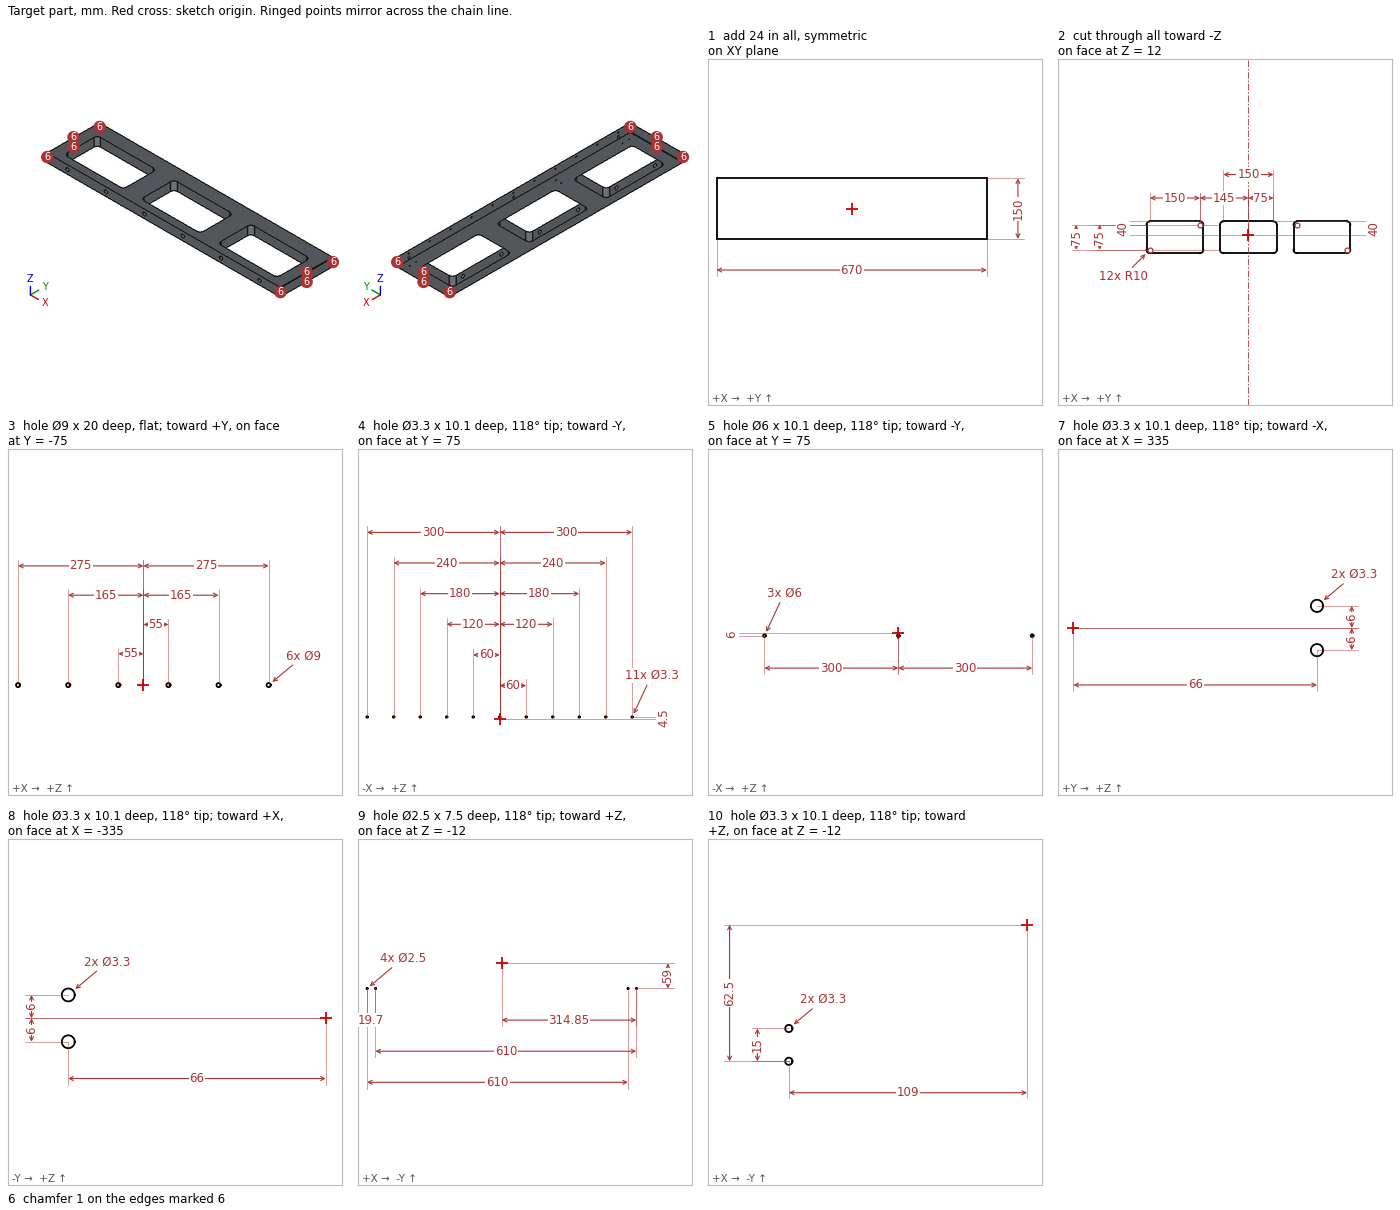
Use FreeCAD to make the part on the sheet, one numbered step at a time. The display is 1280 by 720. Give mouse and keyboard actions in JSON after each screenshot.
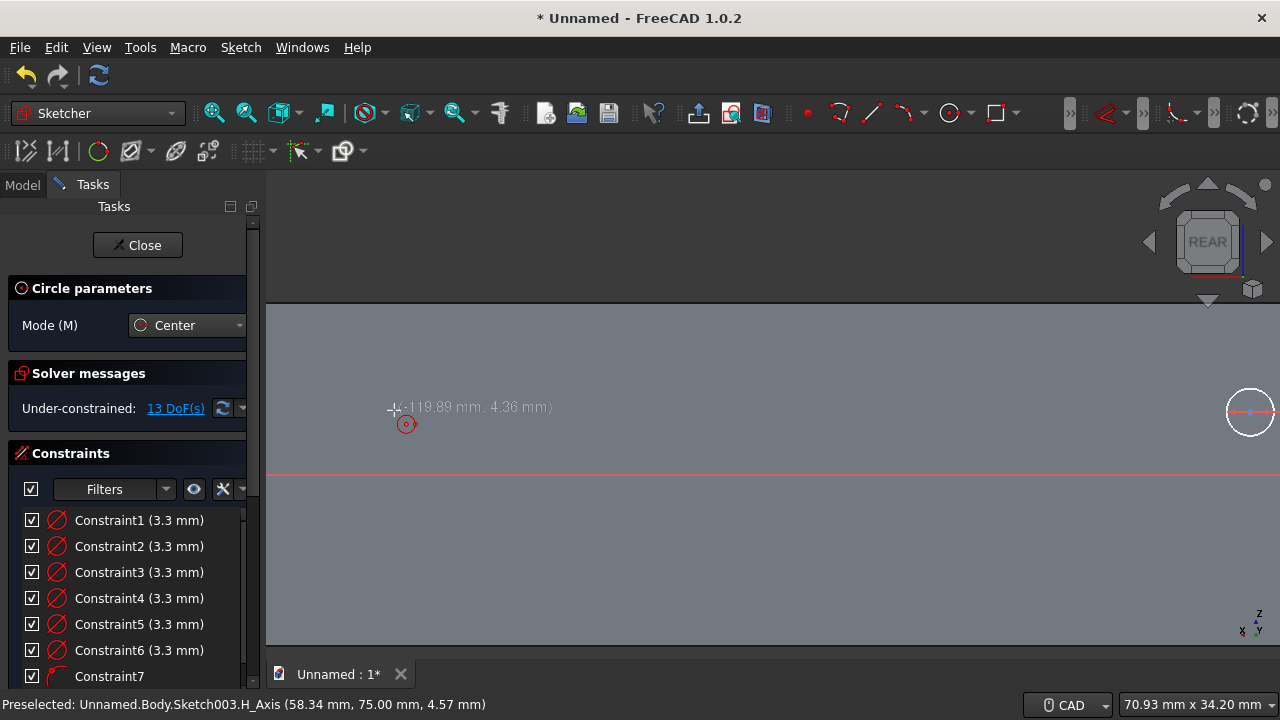
{"action": "scroll", "coordinate": [614, 413], "scroll_direction": "down", "scroll_amount": 14}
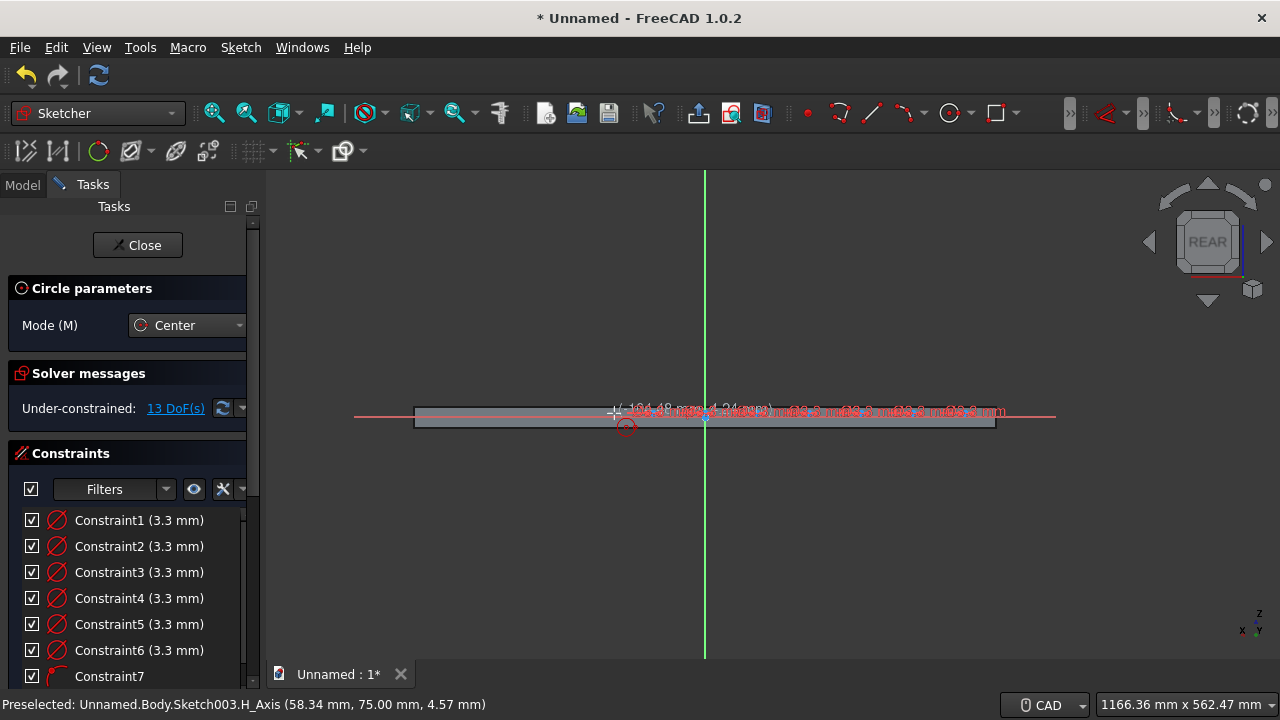
{"action": "scroll", "coordinate": [601, 413], "scroll_direction": "up", "scroll_amount": 8}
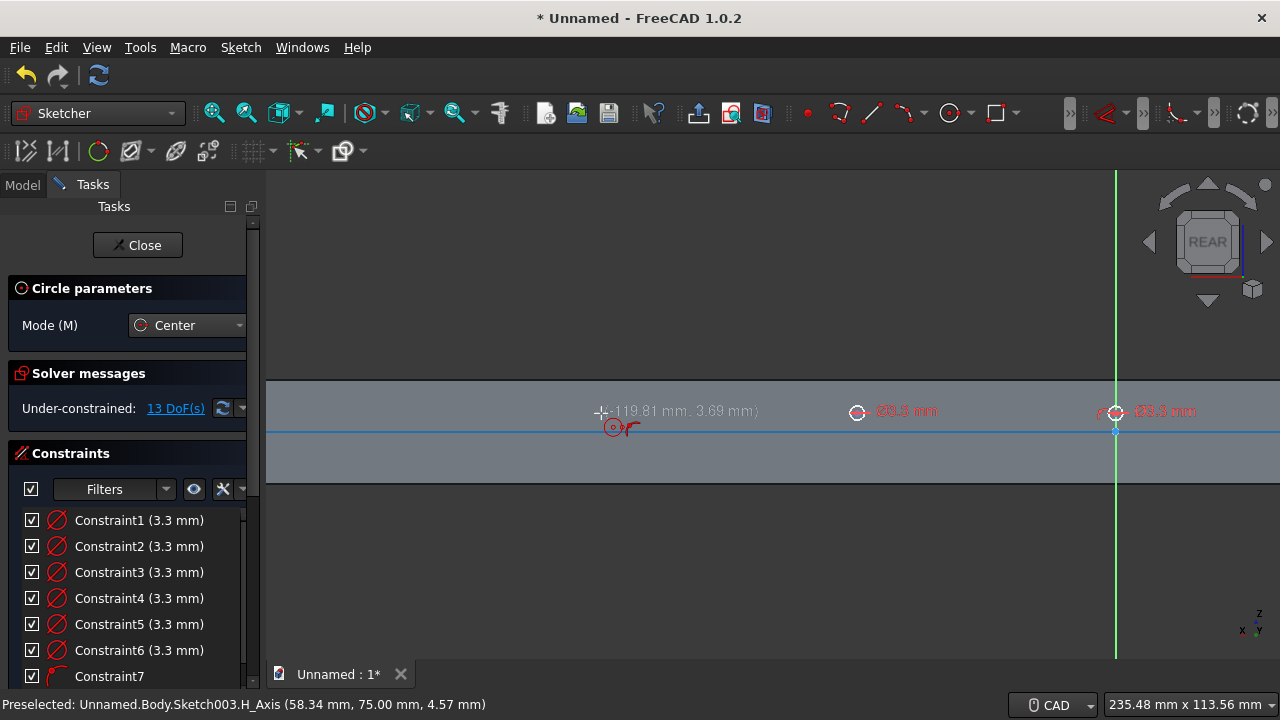
{"action": "left_click", "coordinate": [599, 413]}
{"action": "mouse_move", "coordinate": [604, 407]}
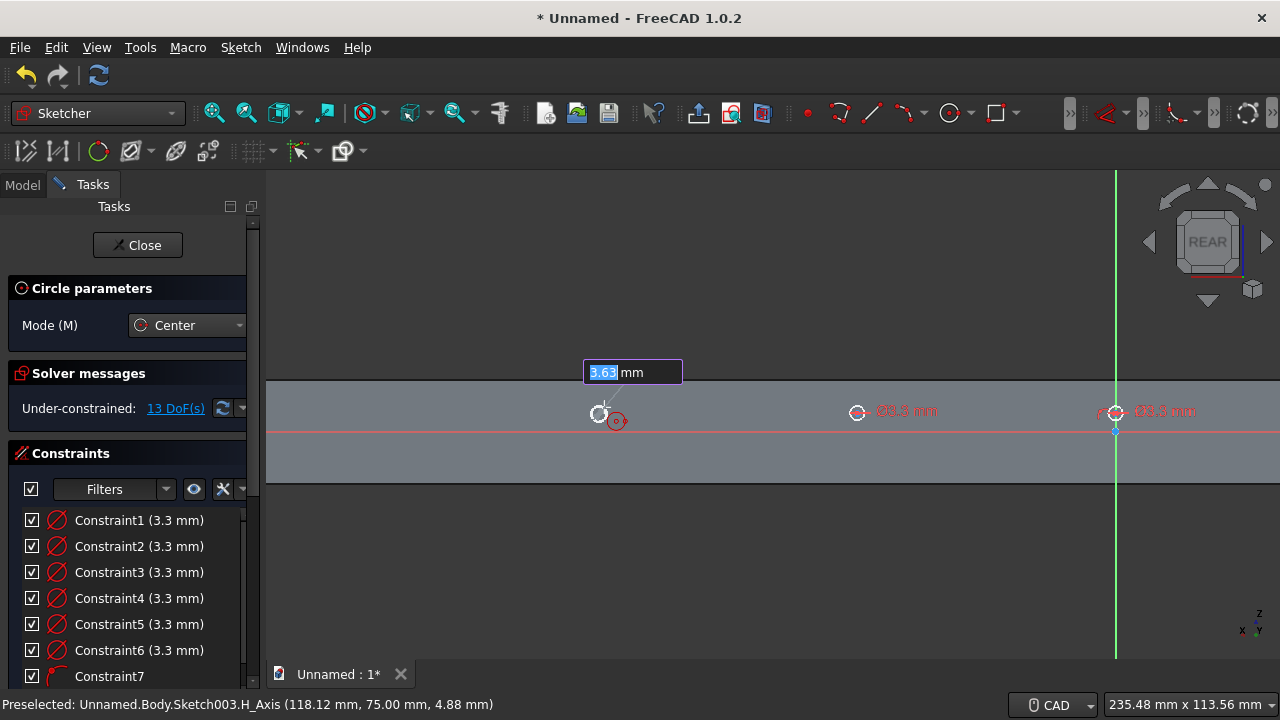
{"action": "type", "text": "3.3"}
{"action": "key", "text": "Return"}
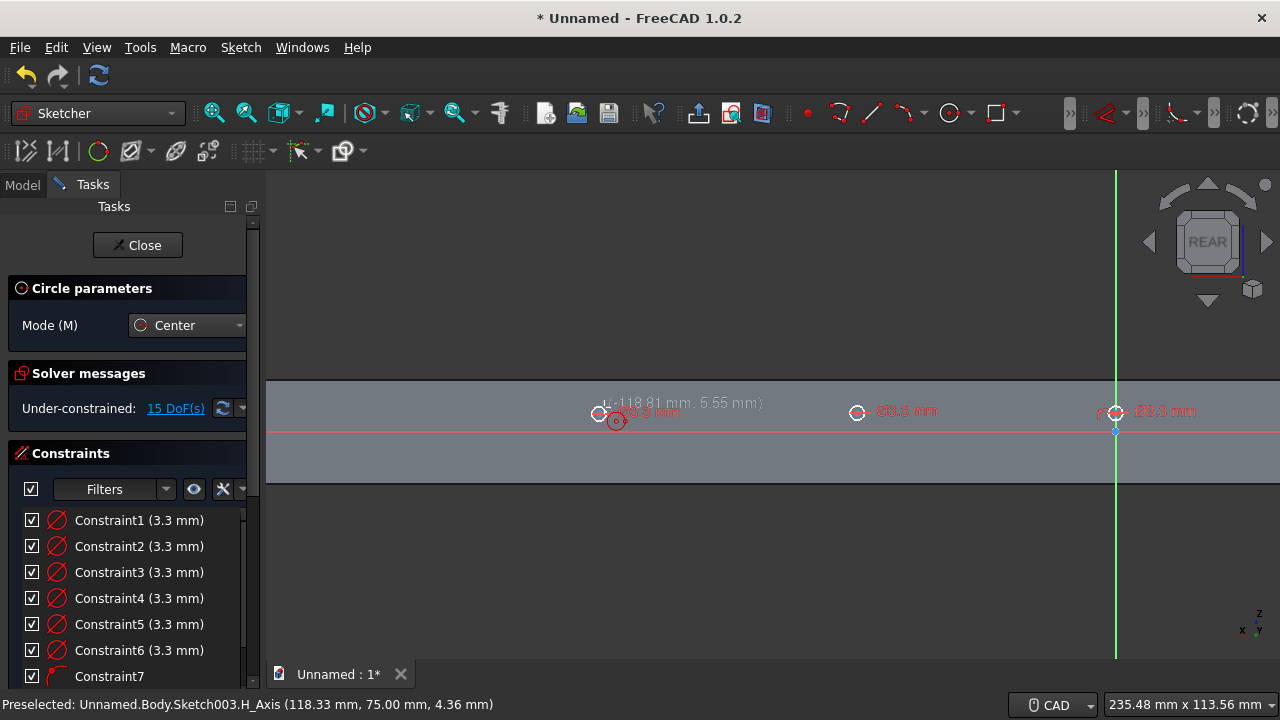
{"action": "scroll", "coordinate": [341, 413], "scroll_direction": "up", "scroll_amount": 6}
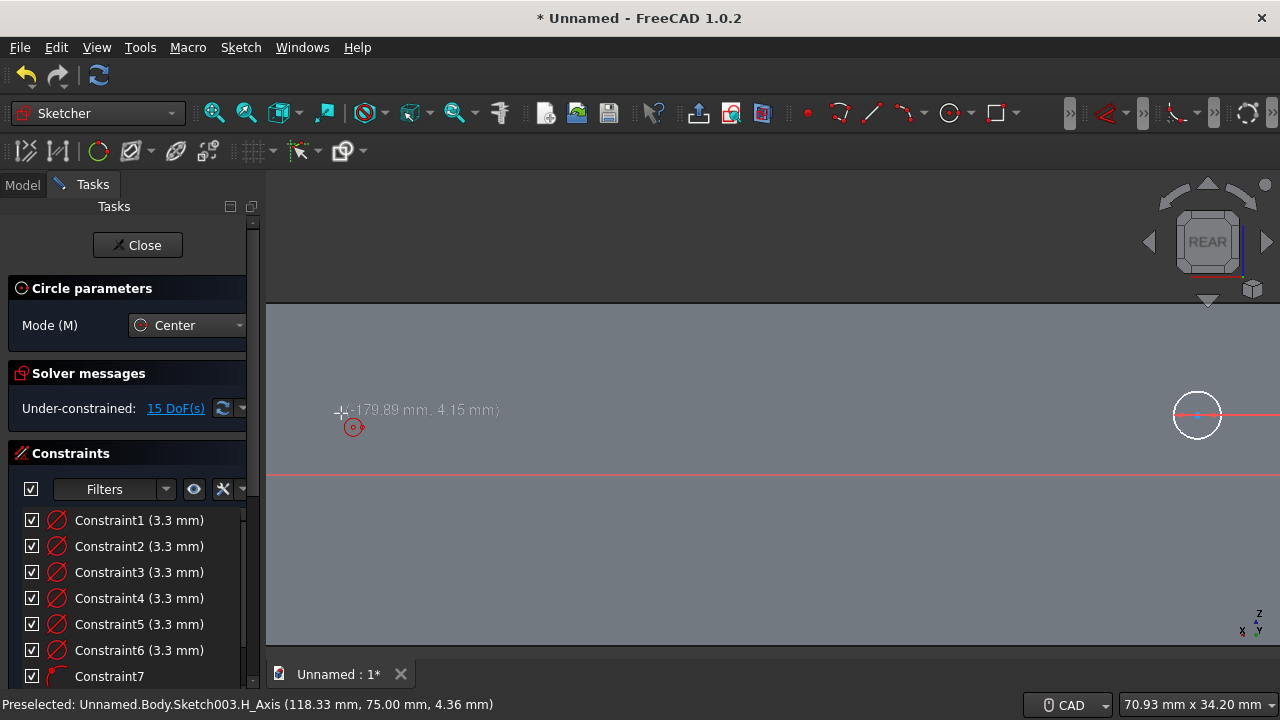
{"action": "scroll", "coordinate": [562, 413], "scroll_direction": "down", "scroll_amount": 14}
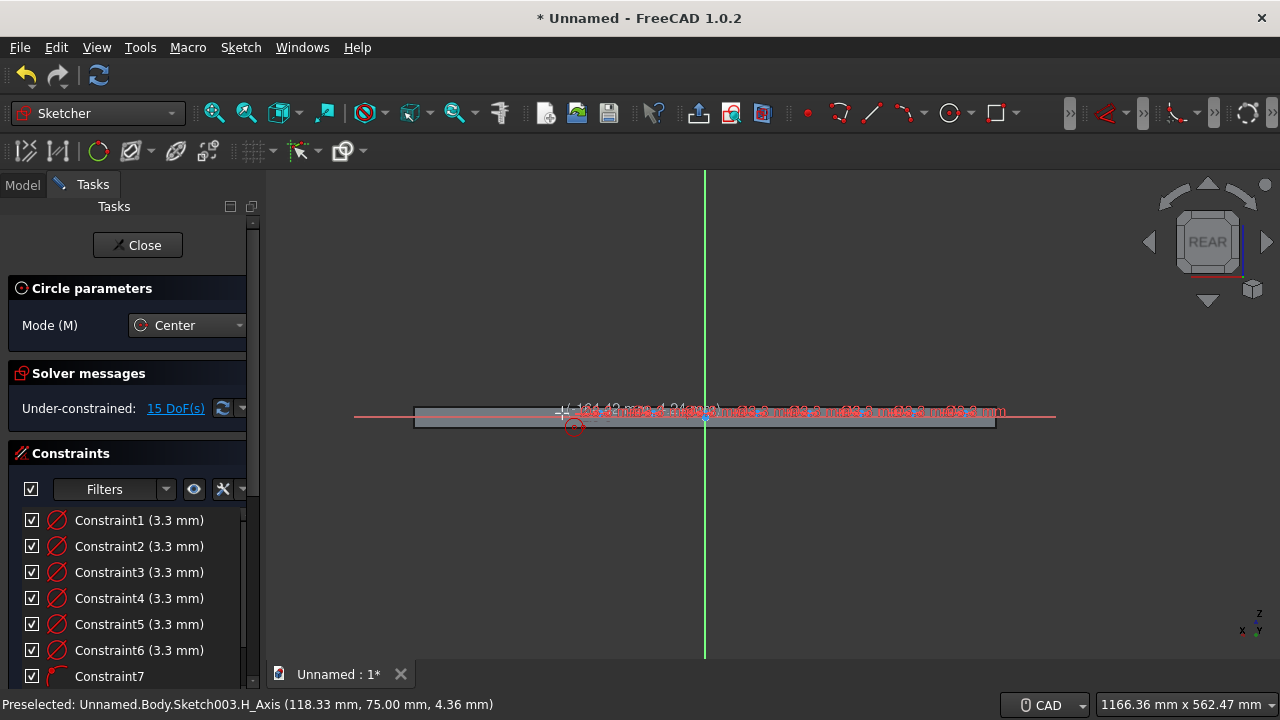
{"action": "scroll", "coordinate": [549, 413], "scroll_direction": "up", "scroll_amount": 8}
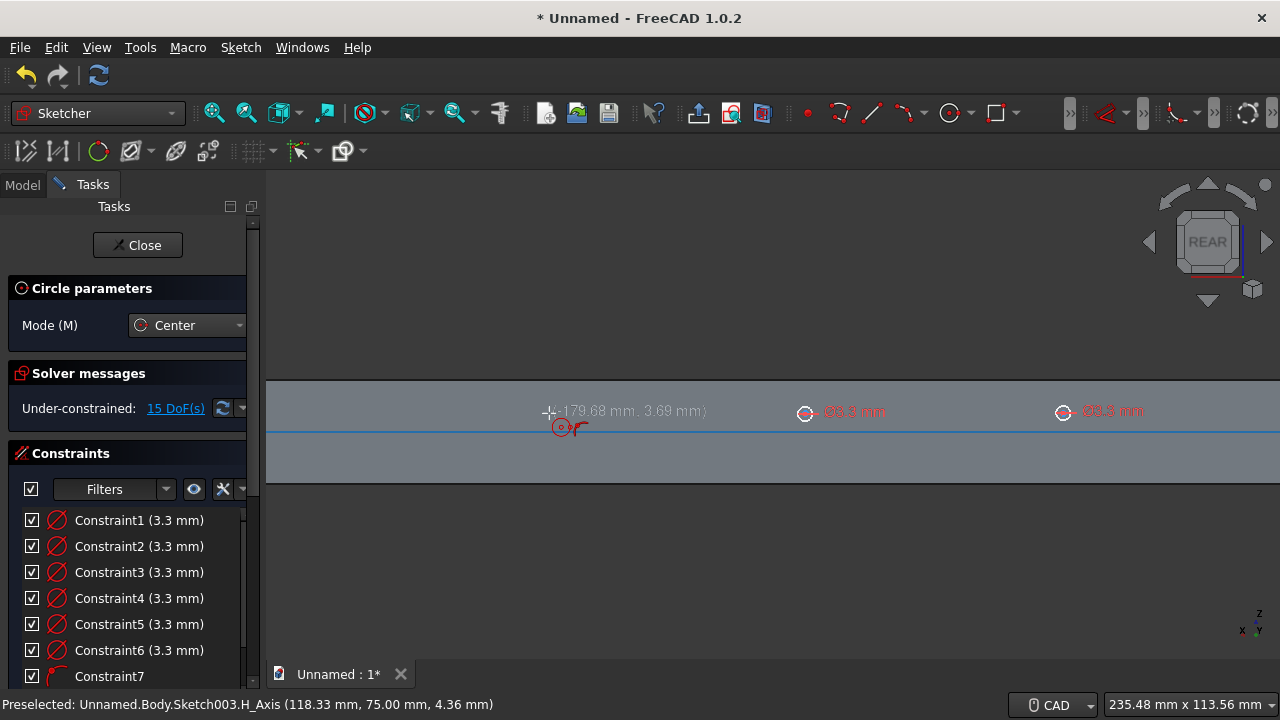
{"action": "left_click", "coordinate": [547, 413]}
{"action": "mouse_move", "coordinate": [552, 407]}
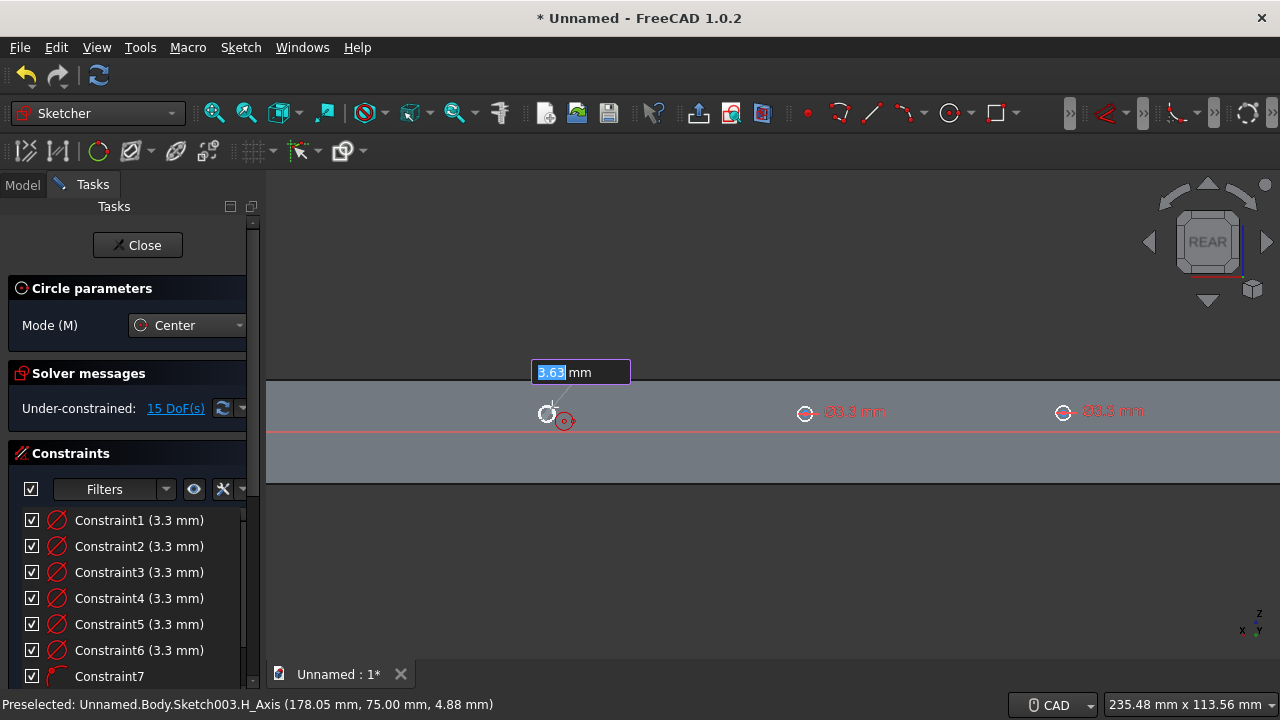
{"action": "type", "text": "3.3"}
{"action": "key", "text": "Return"}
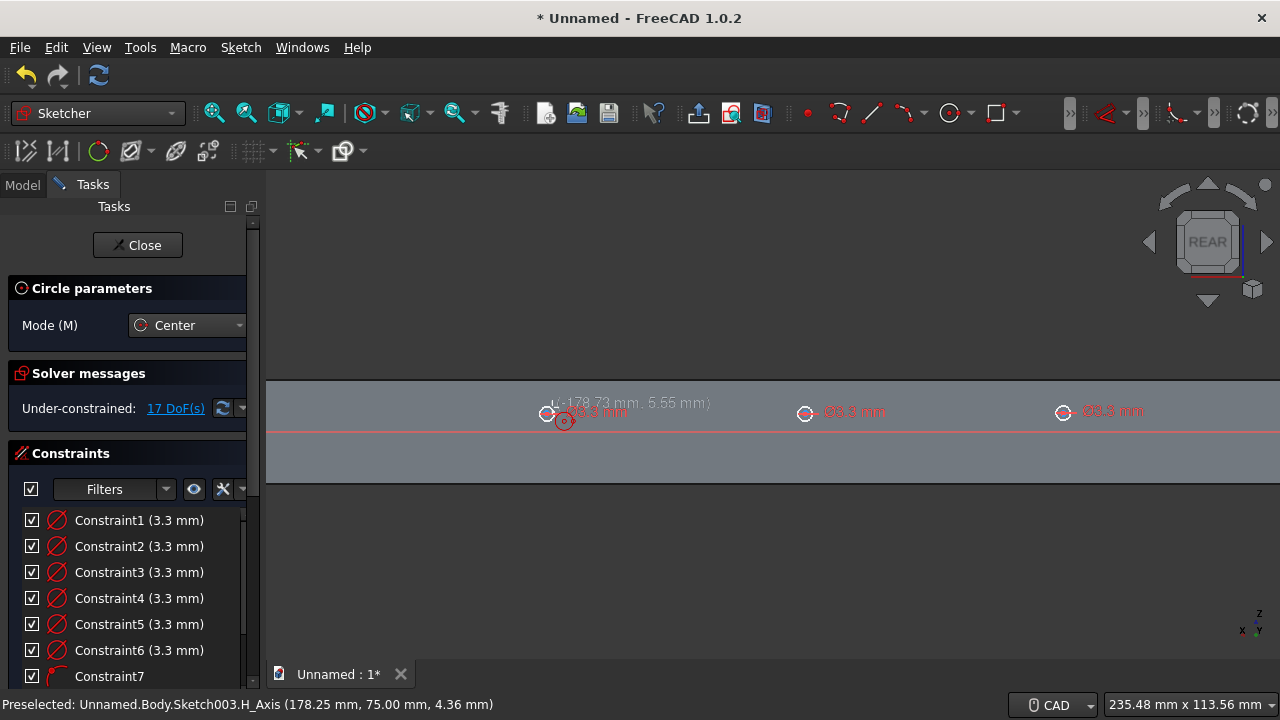
{"action": "scroll", "coordinate": [548, 413], "scroll_direction": "down", "scroll_amount": 8}